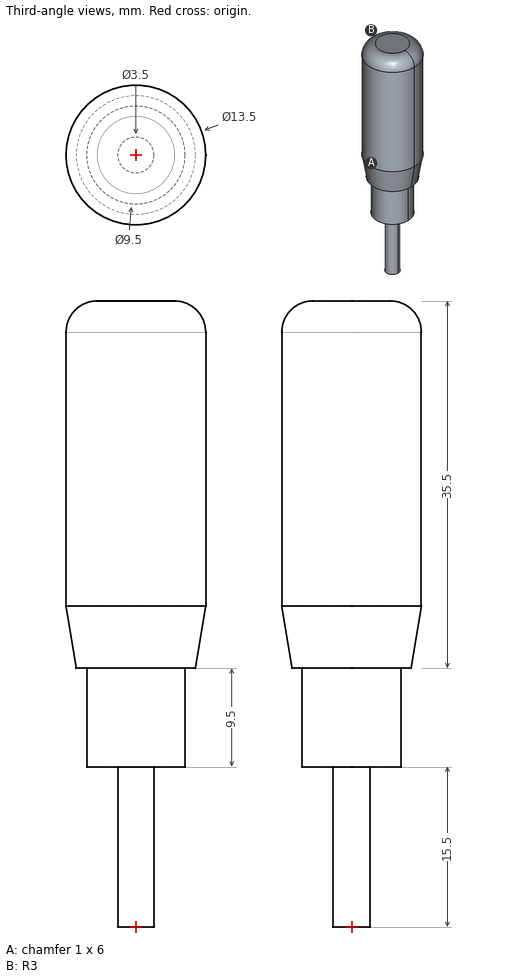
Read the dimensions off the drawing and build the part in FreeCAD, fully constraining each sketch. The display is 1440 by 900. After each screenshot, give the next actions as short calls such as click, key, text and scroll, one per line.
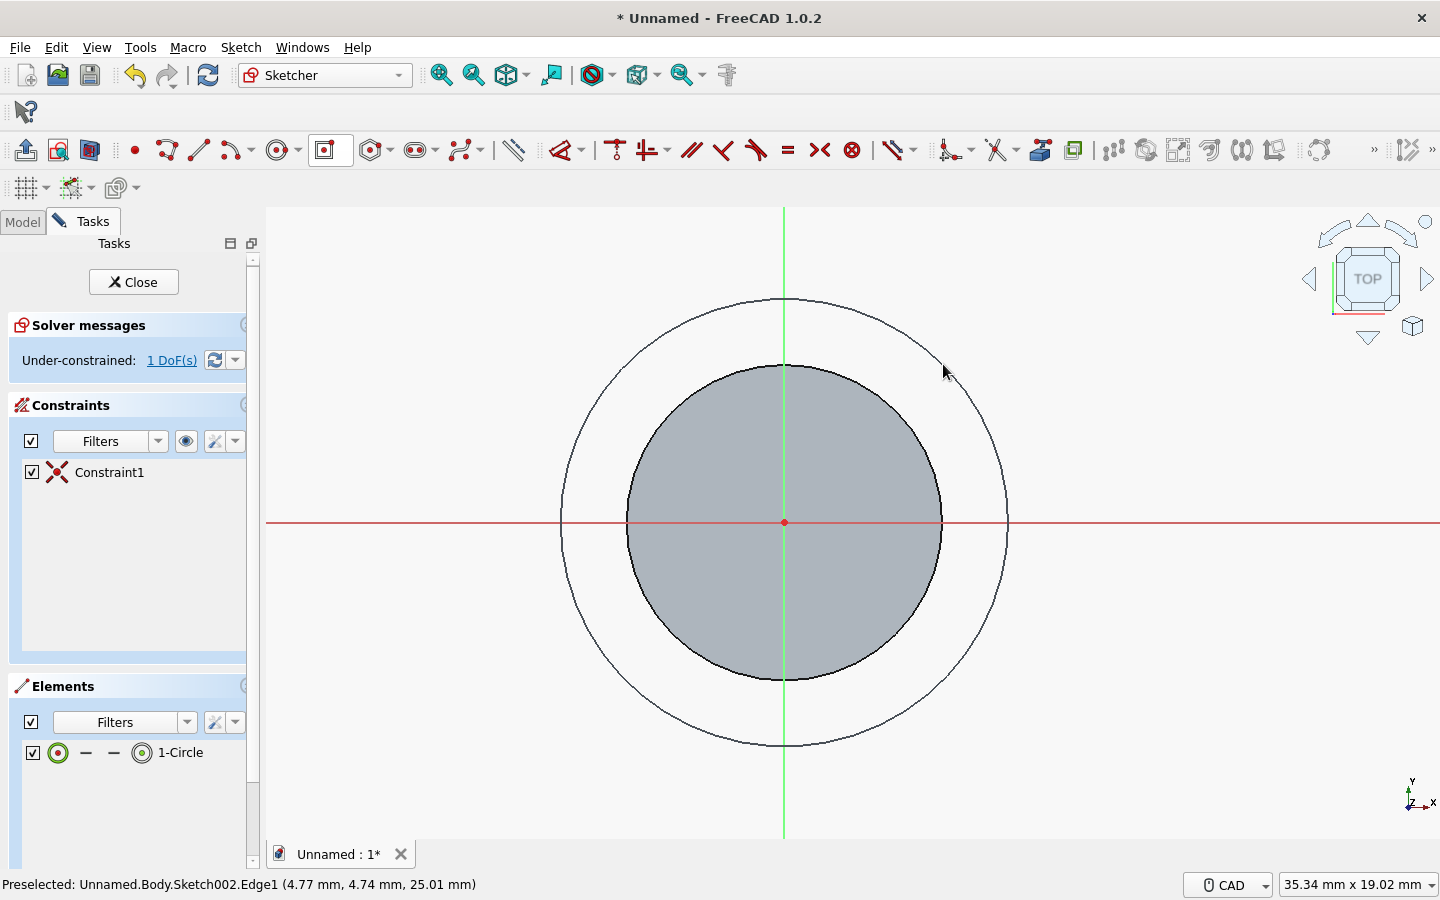
click(560, 150)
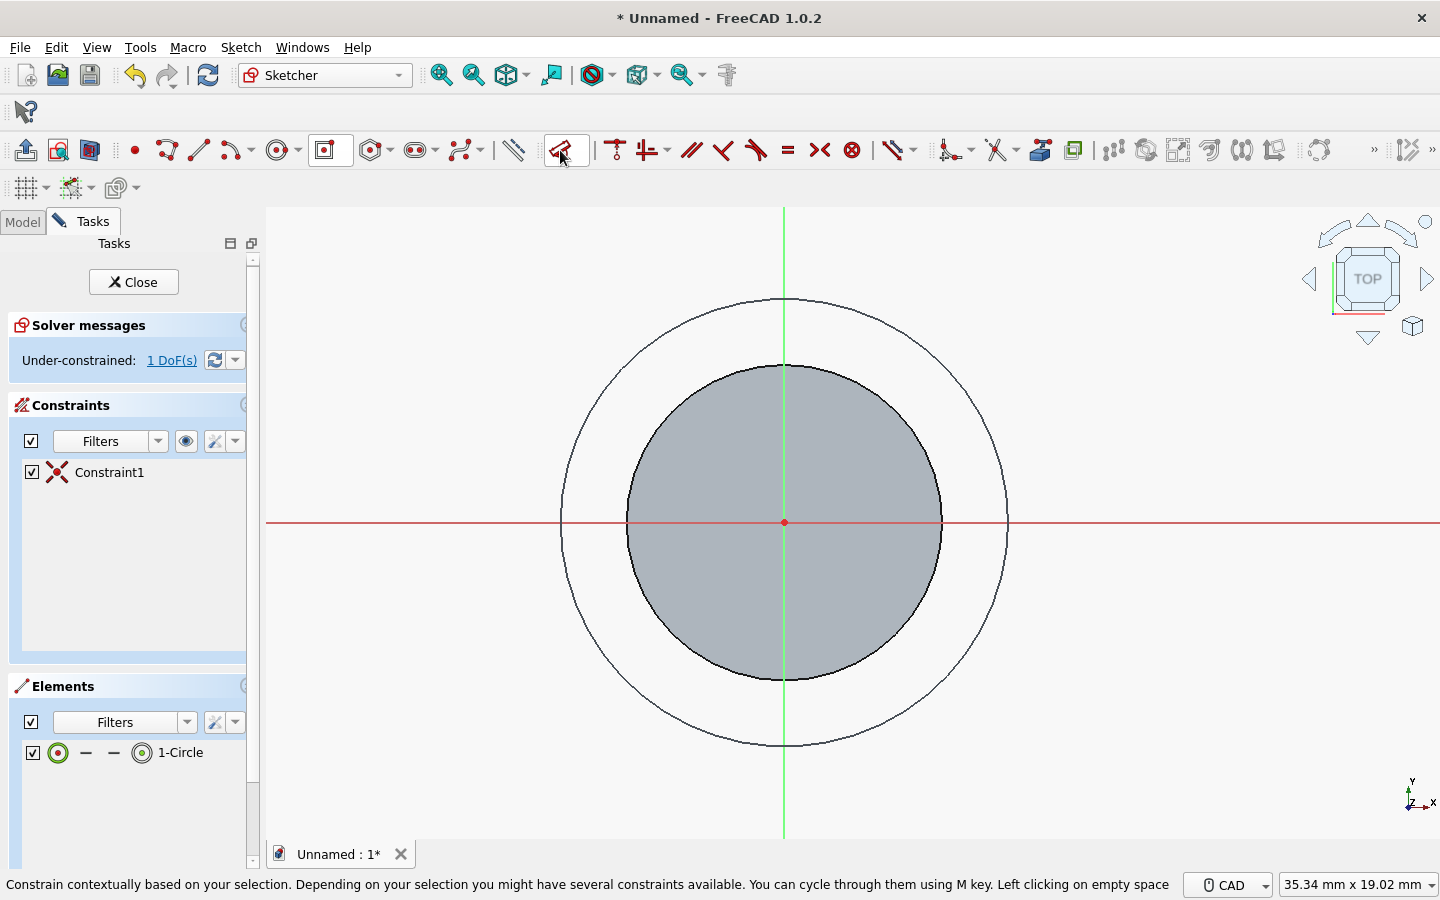
click(942, 364)
click(965, 341)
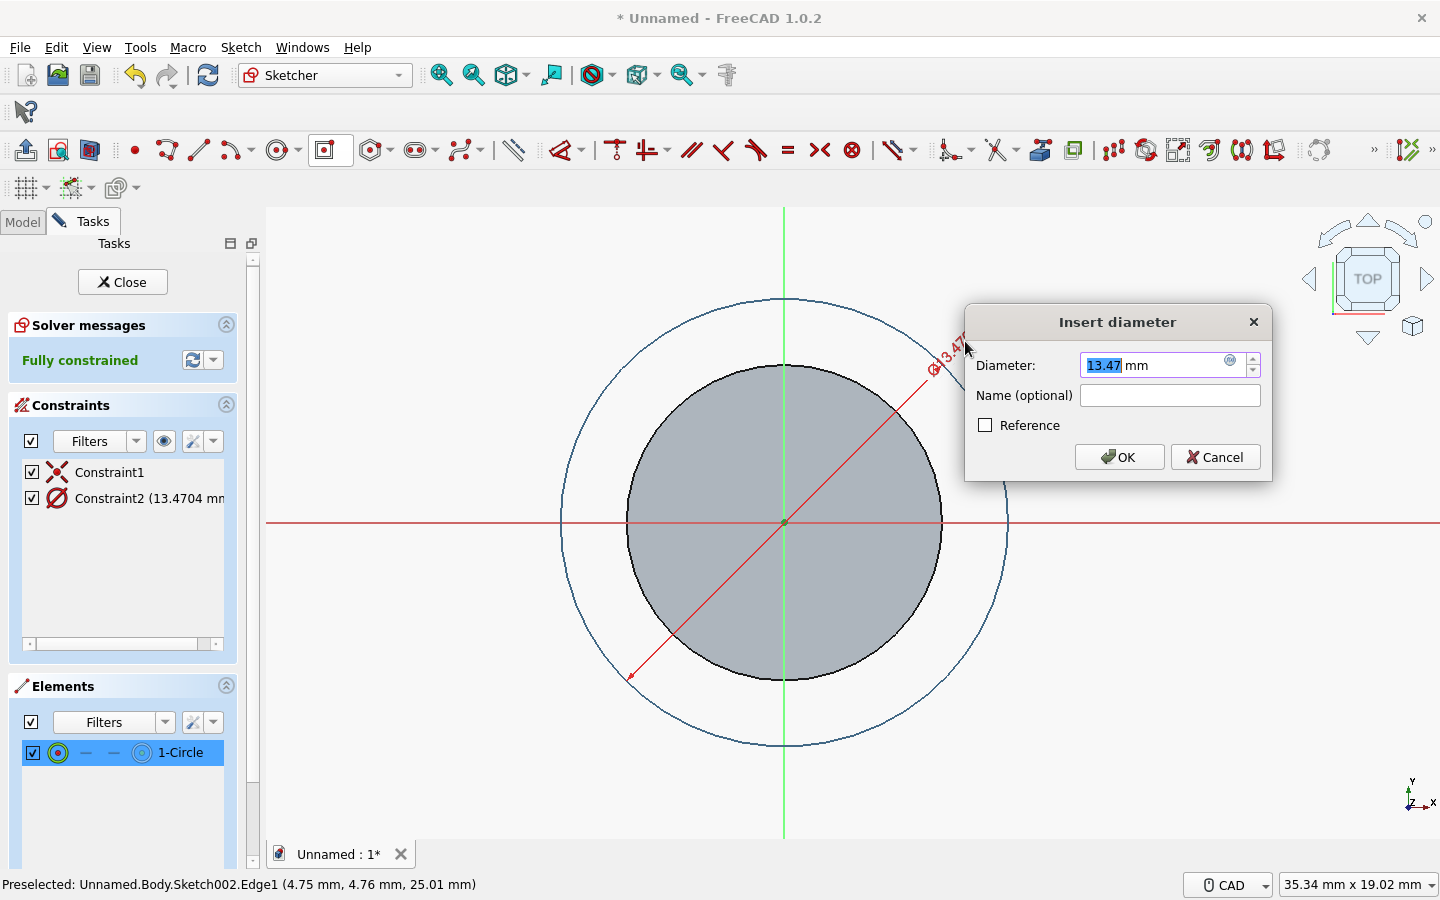
text(13.5)
key(Return)
key(Escape)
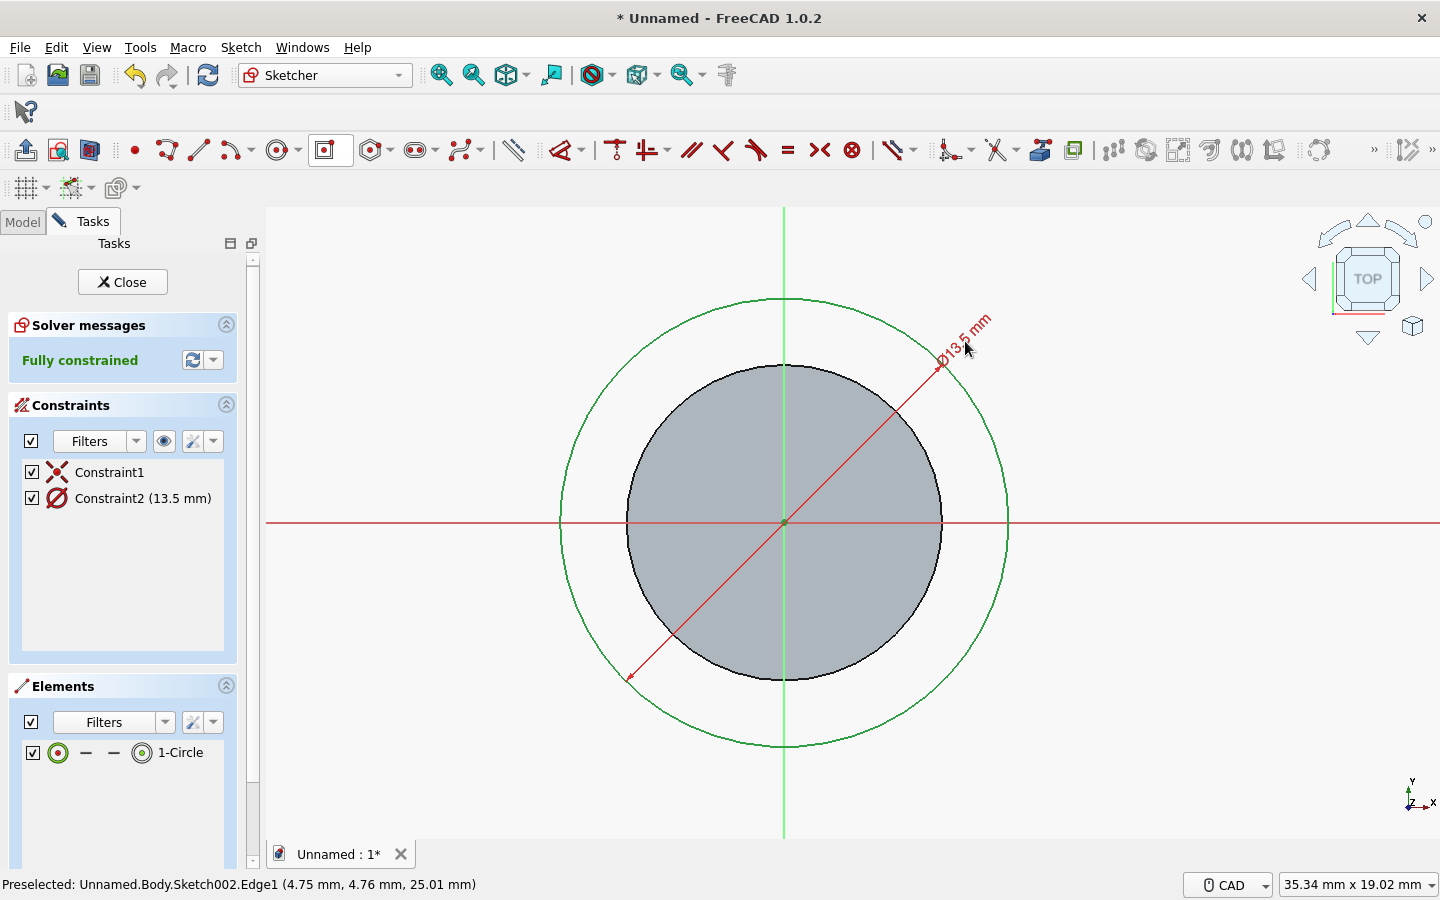
click(123, 282)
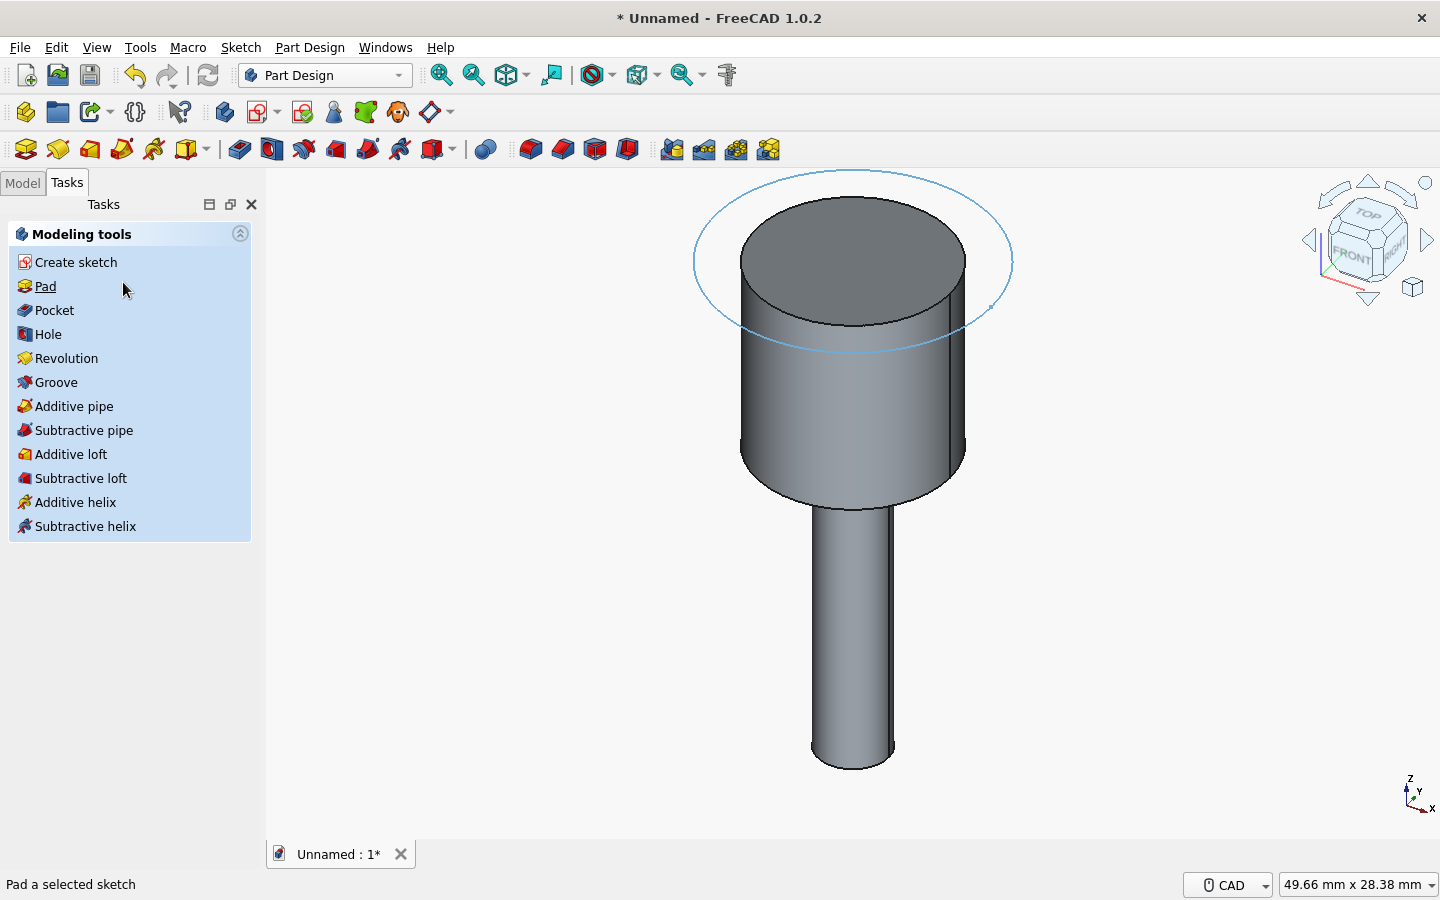
click(26, 150)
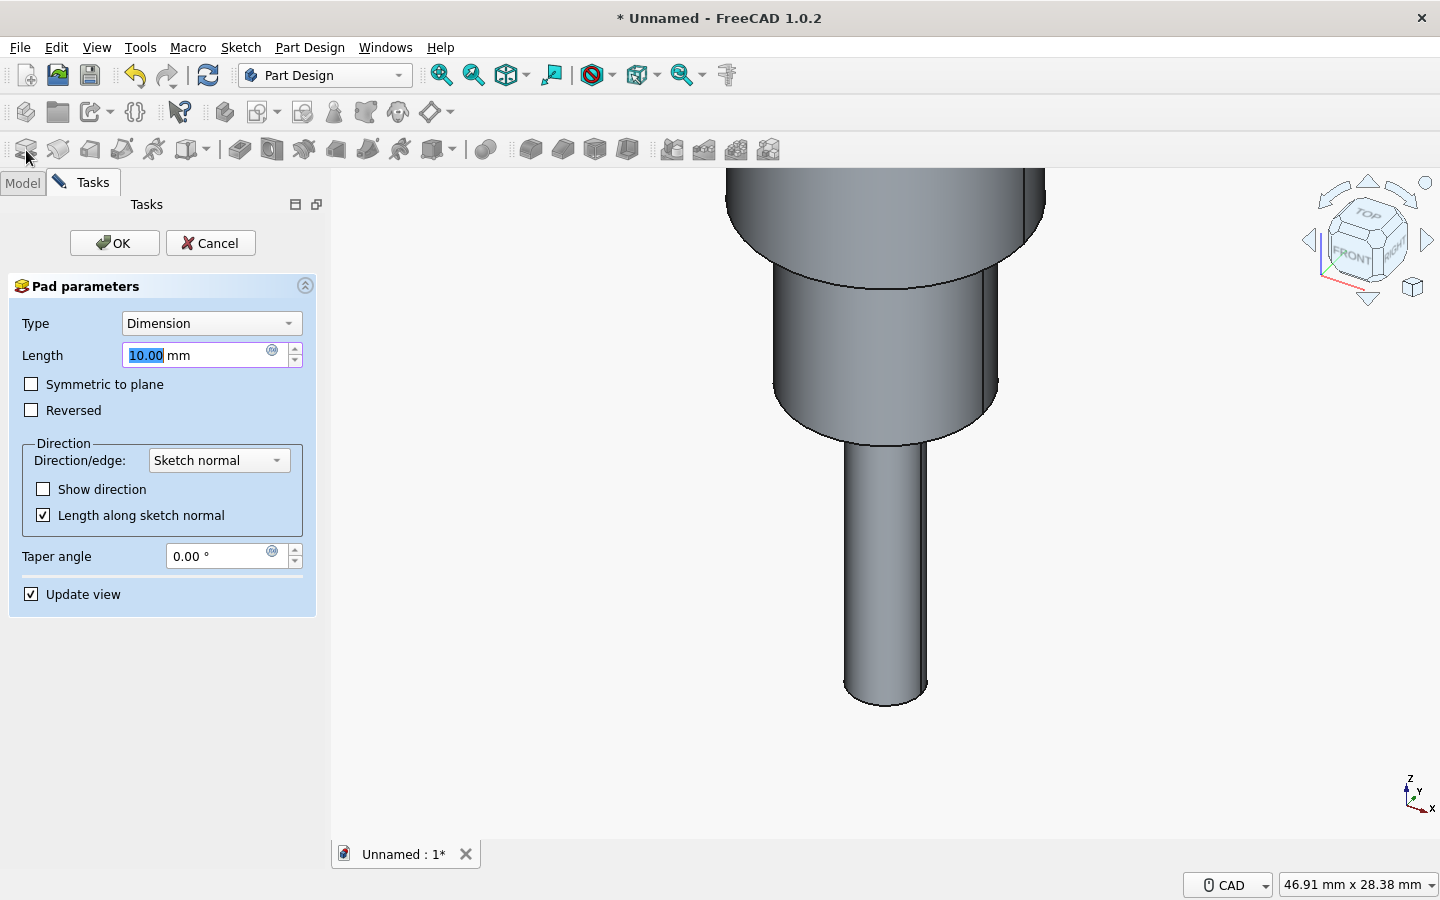
text(35.5)
key(Tab)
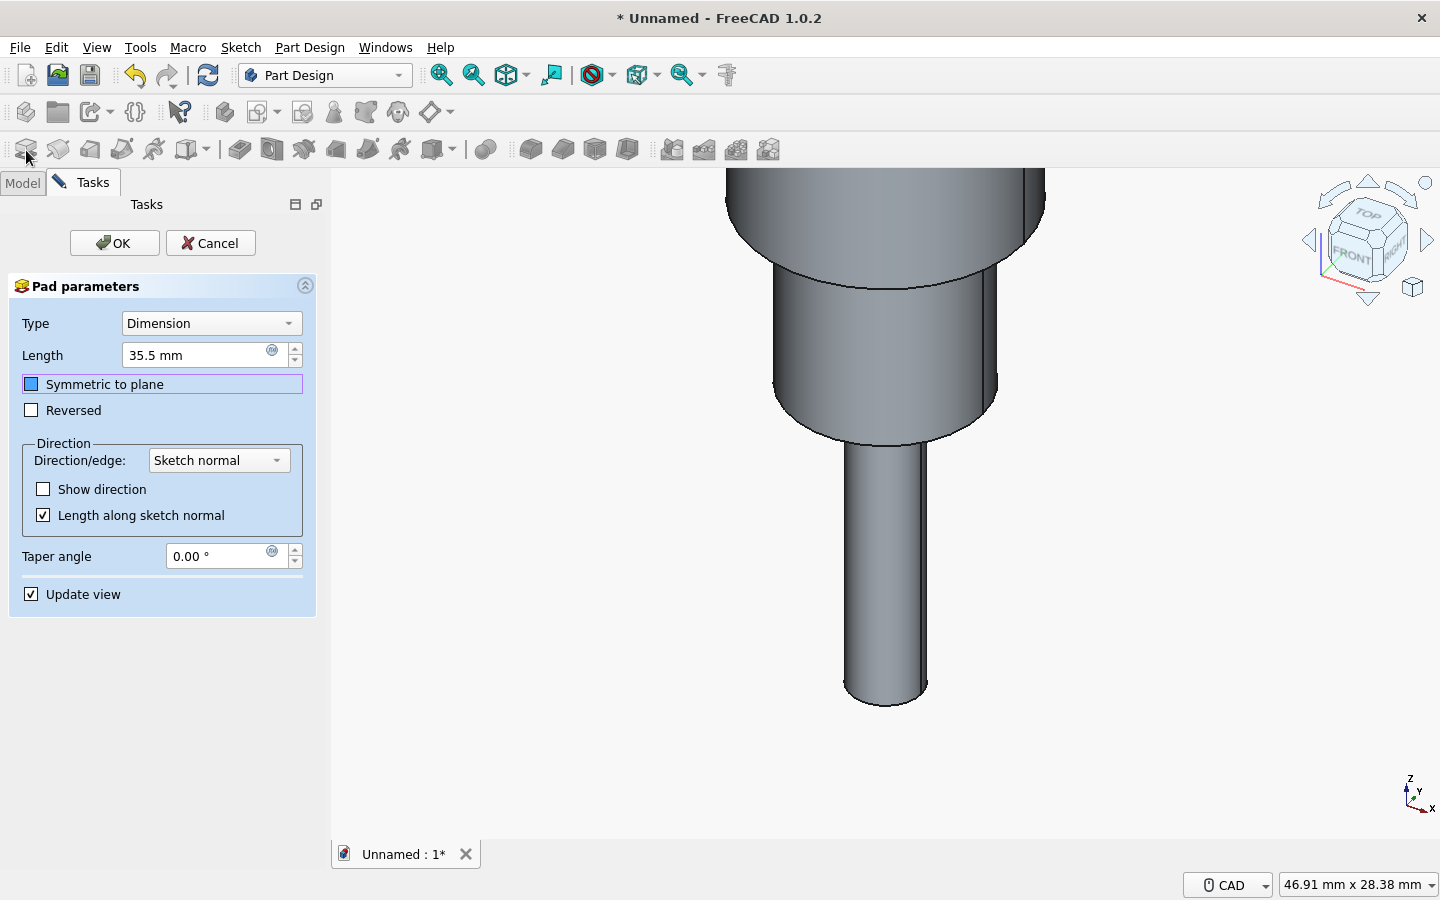
click(115, 243)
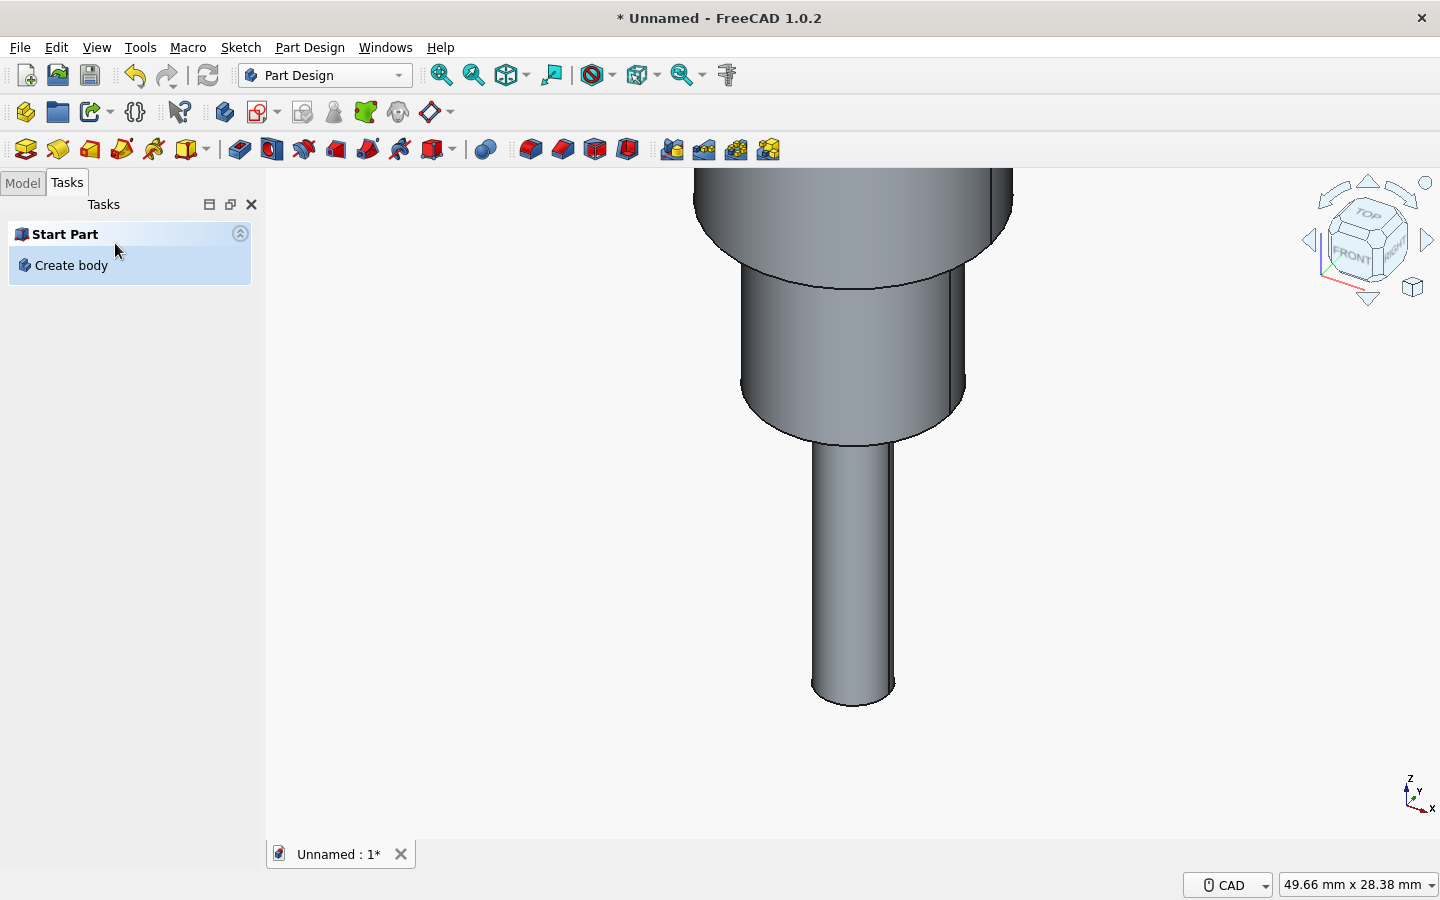
click(442, 76)